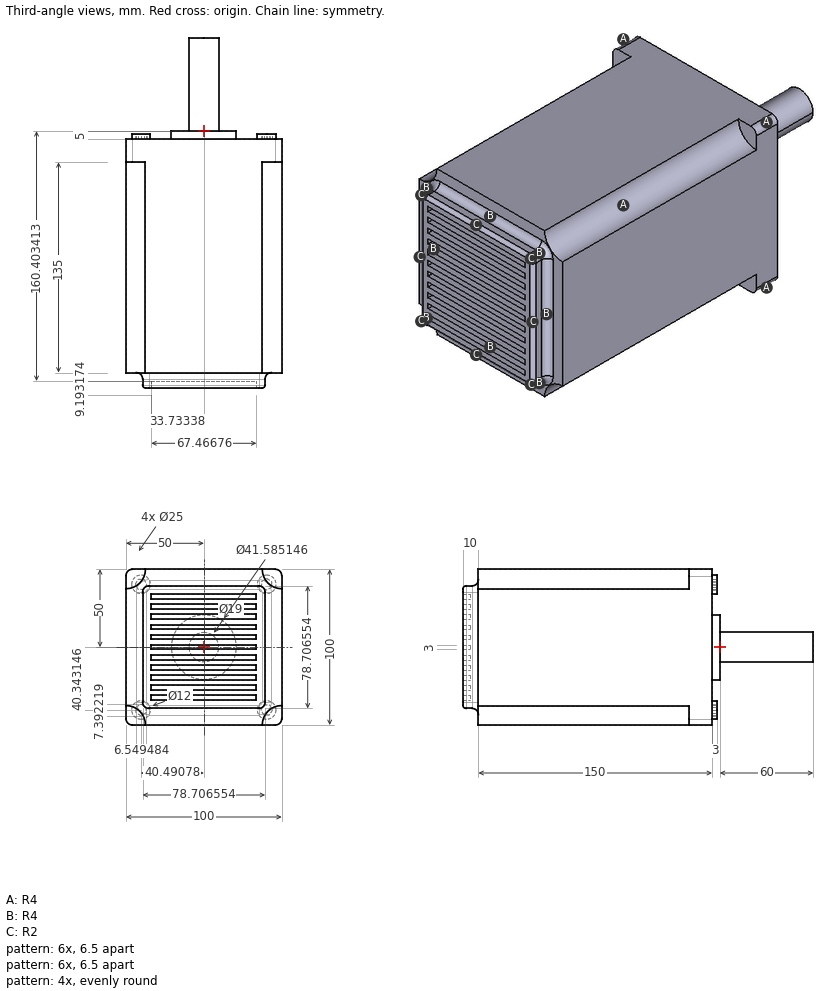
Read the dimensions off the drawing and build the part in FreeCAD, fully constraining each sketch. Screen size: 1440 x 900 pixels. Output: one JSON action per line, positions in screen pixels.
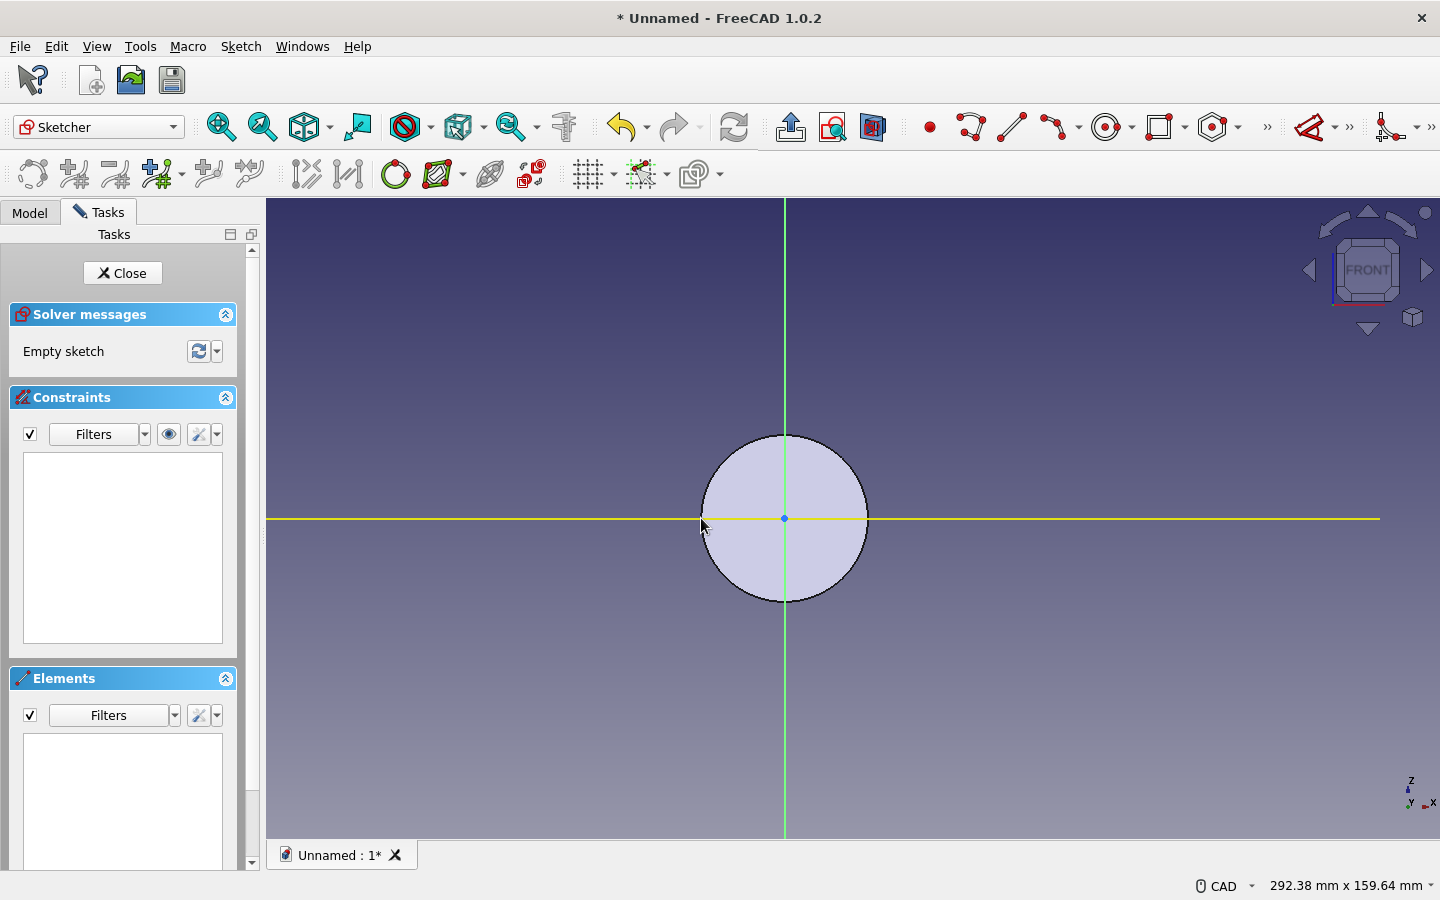
{"action": "left_click", "coordinate": [1184, 128]}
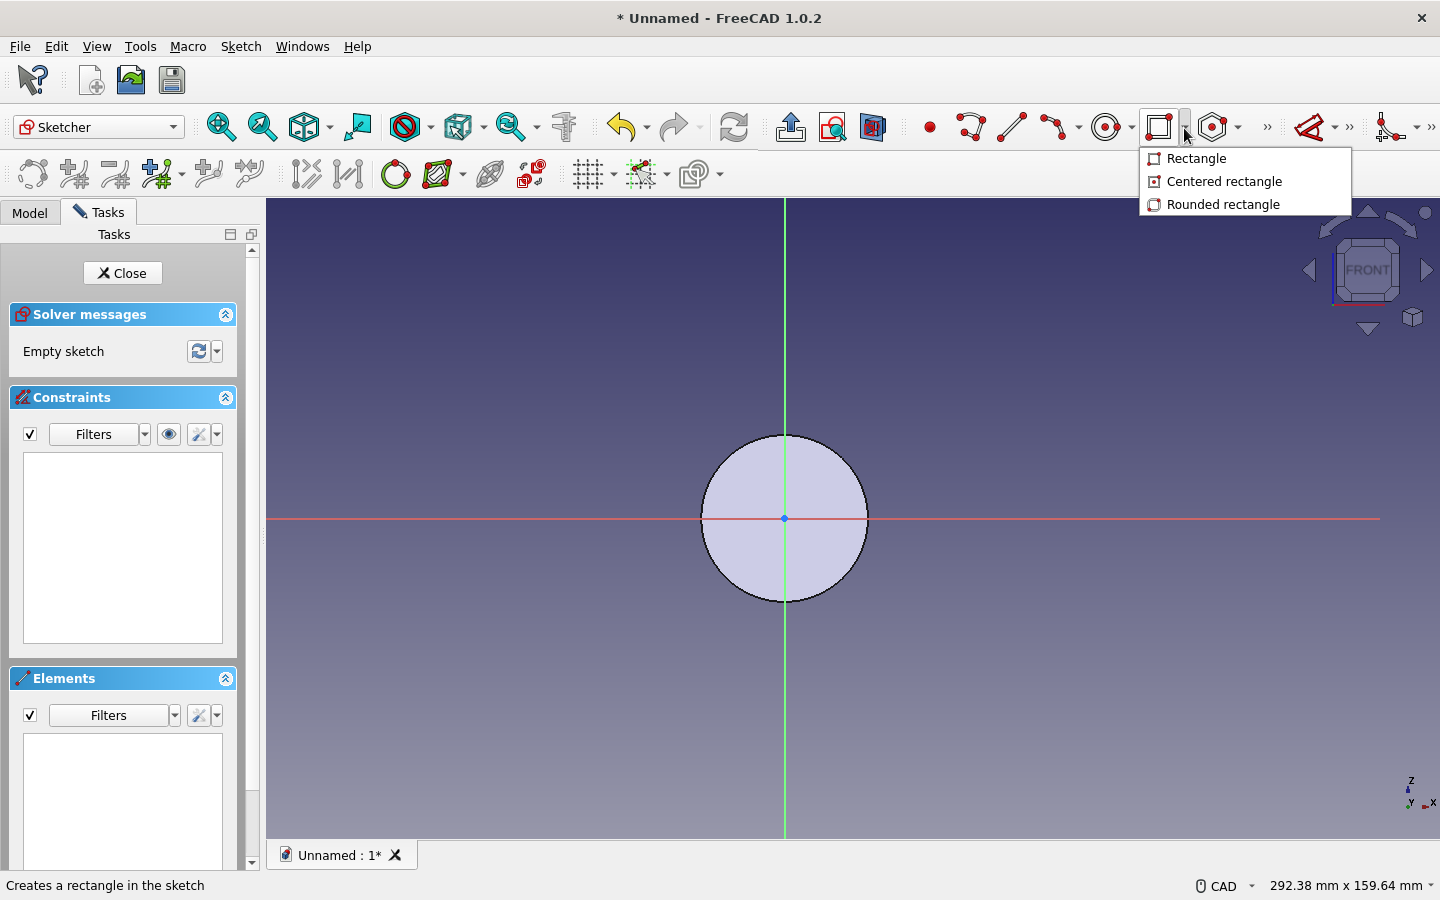
{"action": "left_click", "coordinate": [1246, 182]}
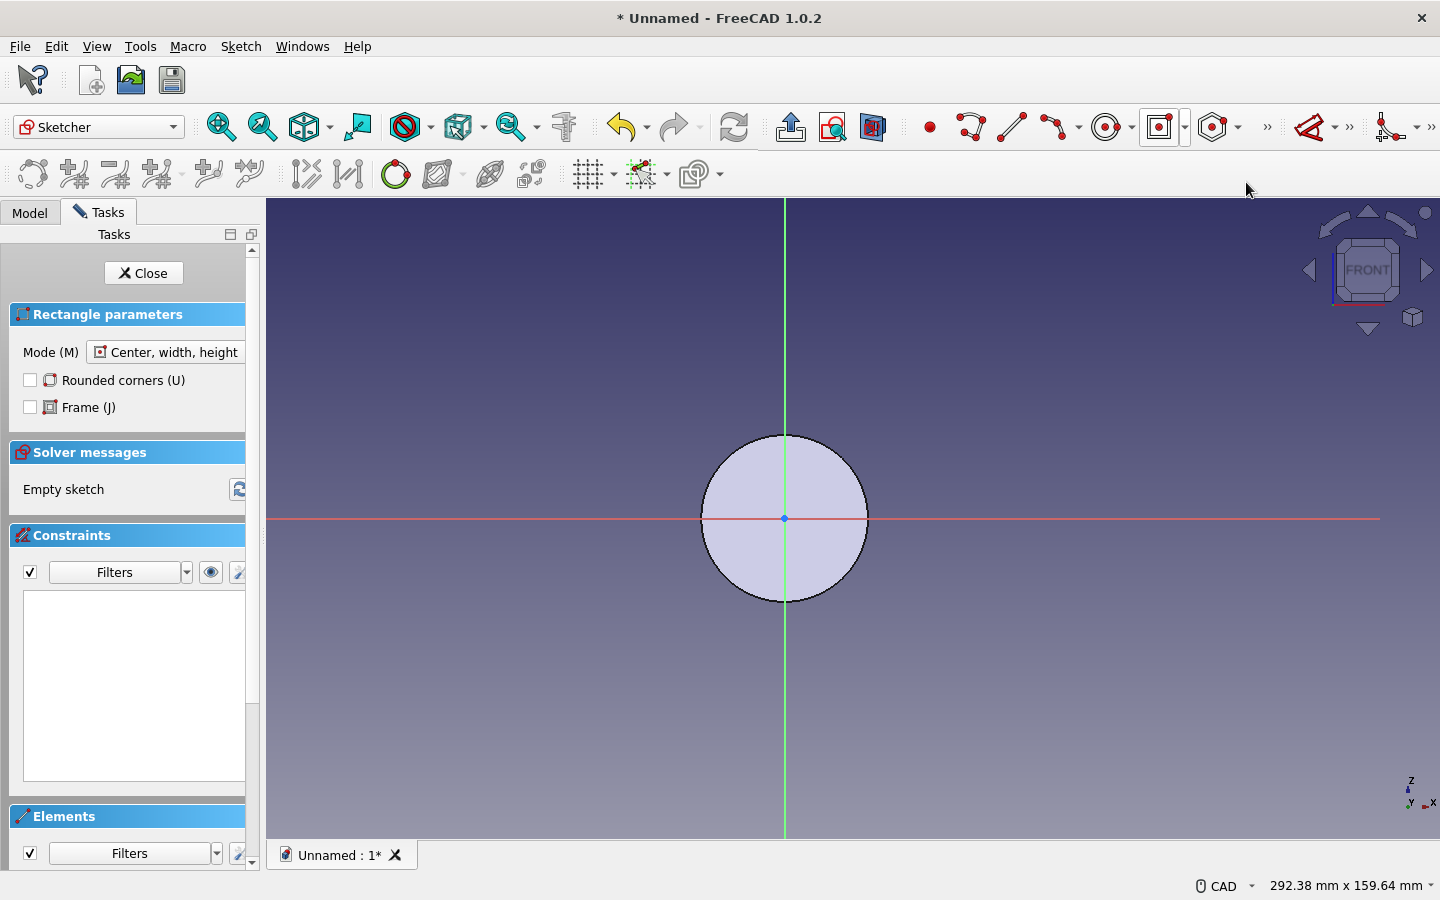
{"action": "left_click", "coordinate": [785, 519]}
{"action": "left_click", "coordinate": [985, 318]}
{"action": "key", "text": "Escape"}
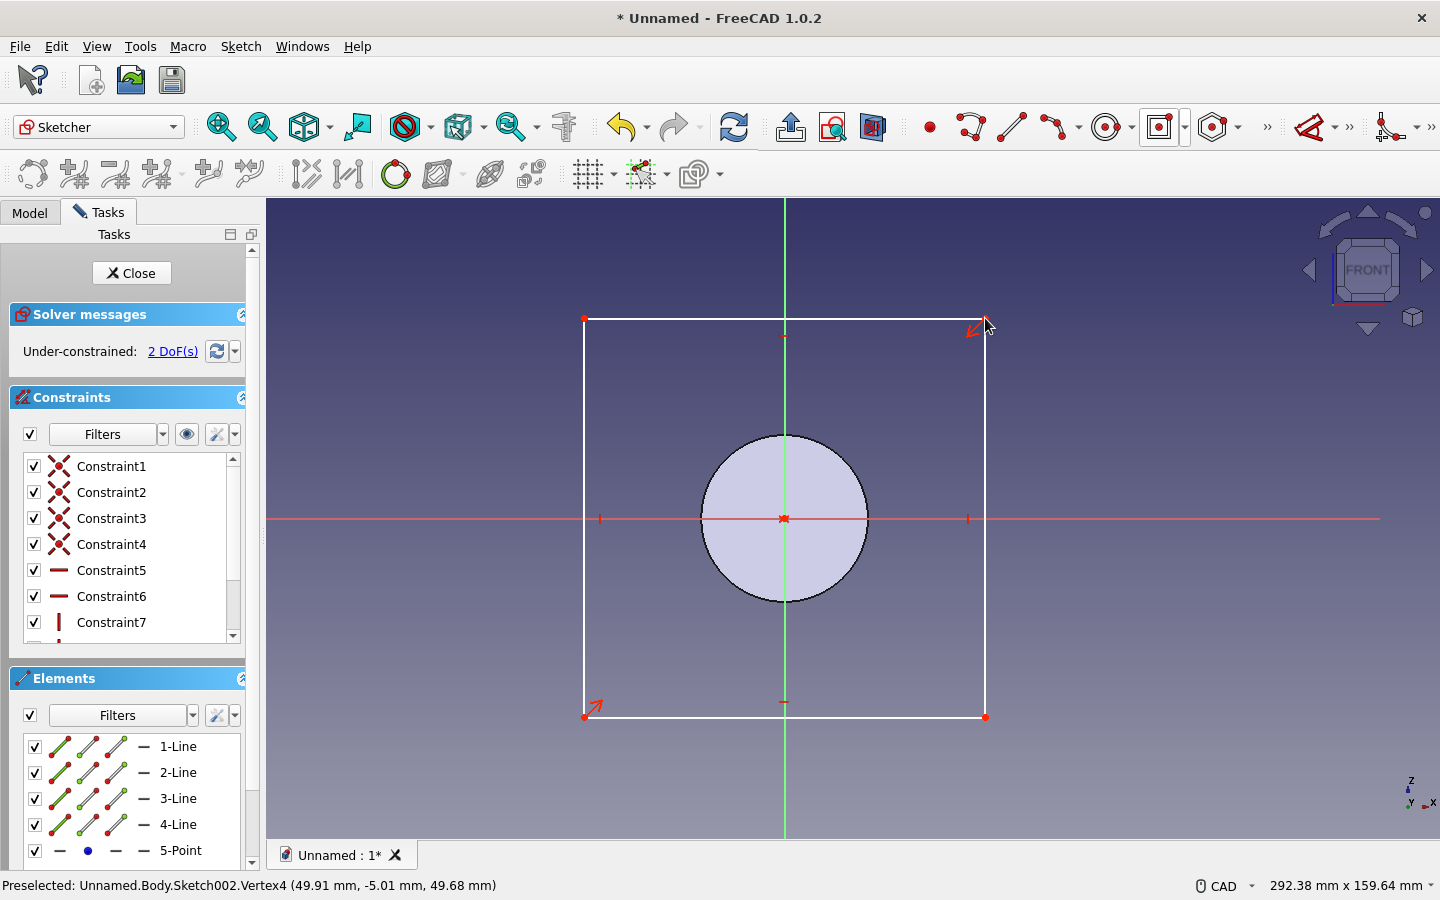
{"action": "left_click", "coordinate": [1308, 128]}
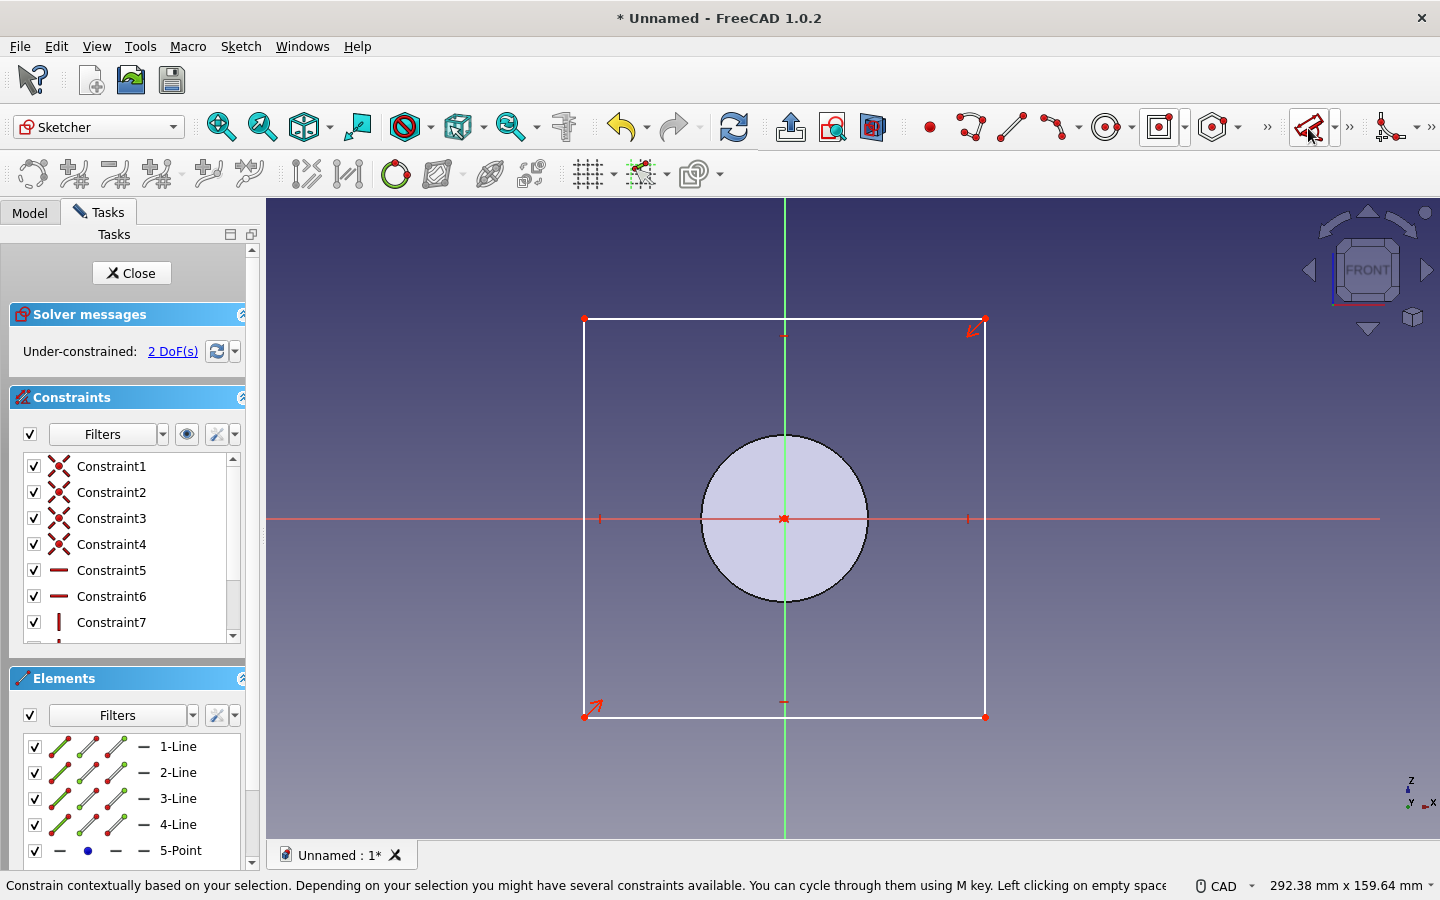
{"action": "left_click", "coordinate": [704, 718]}
{"action": "left_click", "coordinate": [692, 752]}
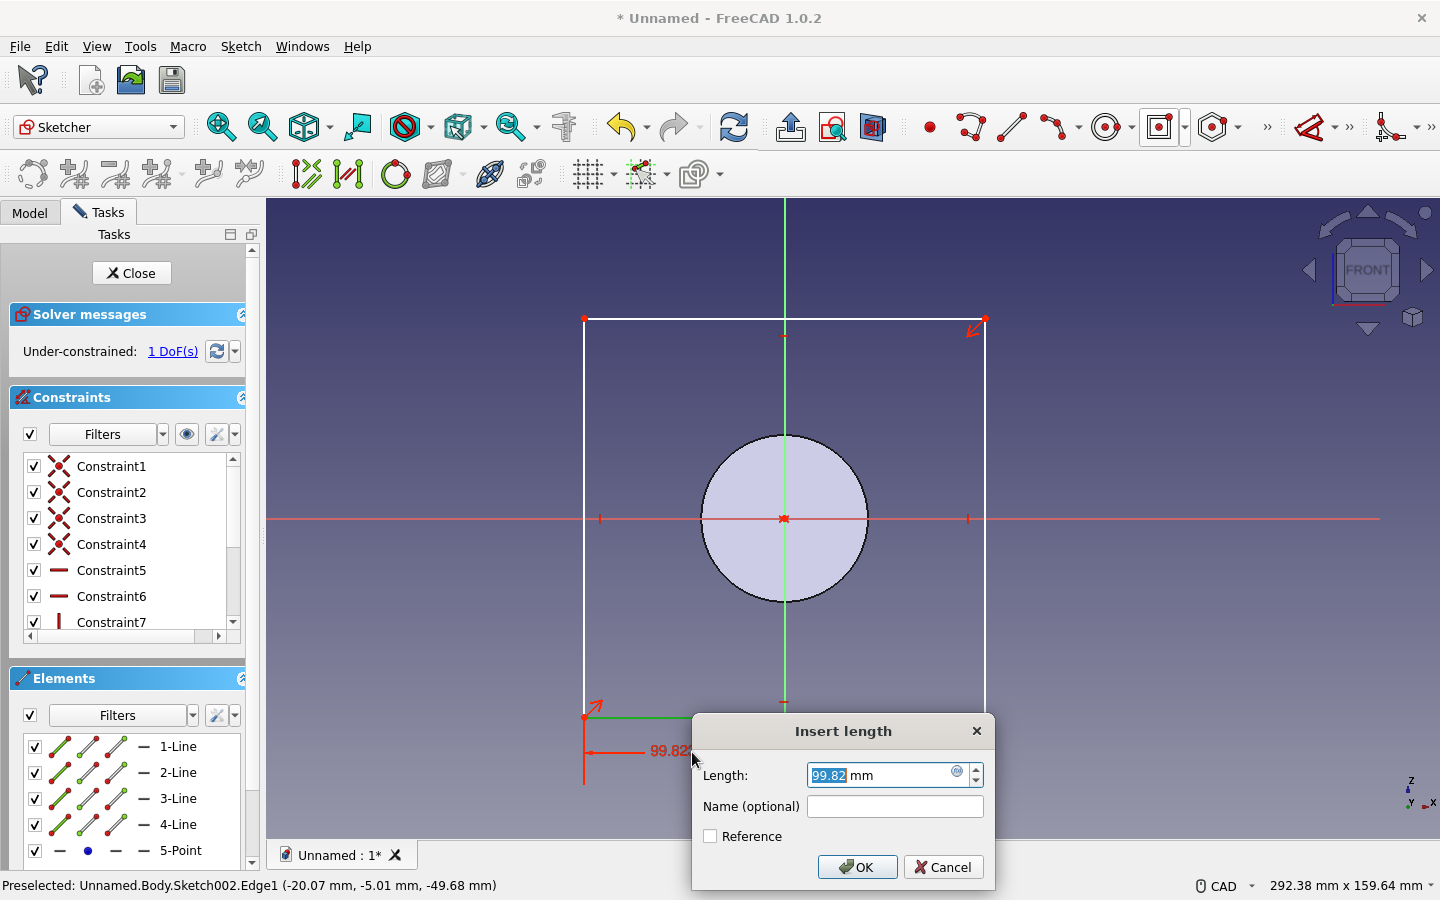
{"action": "type", "text": "100"}
{"action": "key", "text": "Return"}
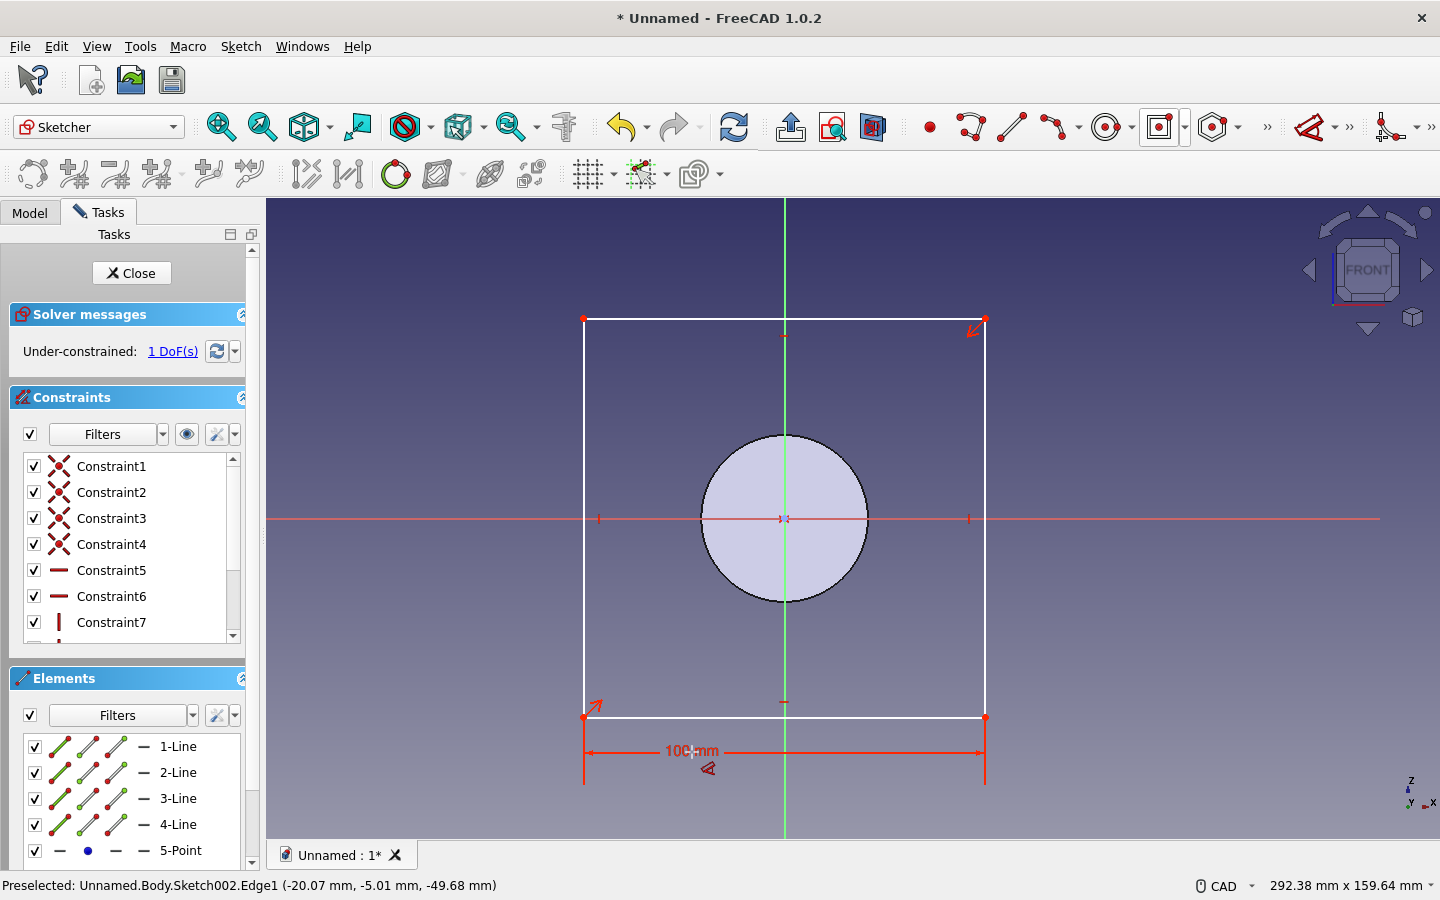
{"action": "left_click", "coordinate": [985, 598]}
{"action": "left_click", "coordinate": [1019, 427]}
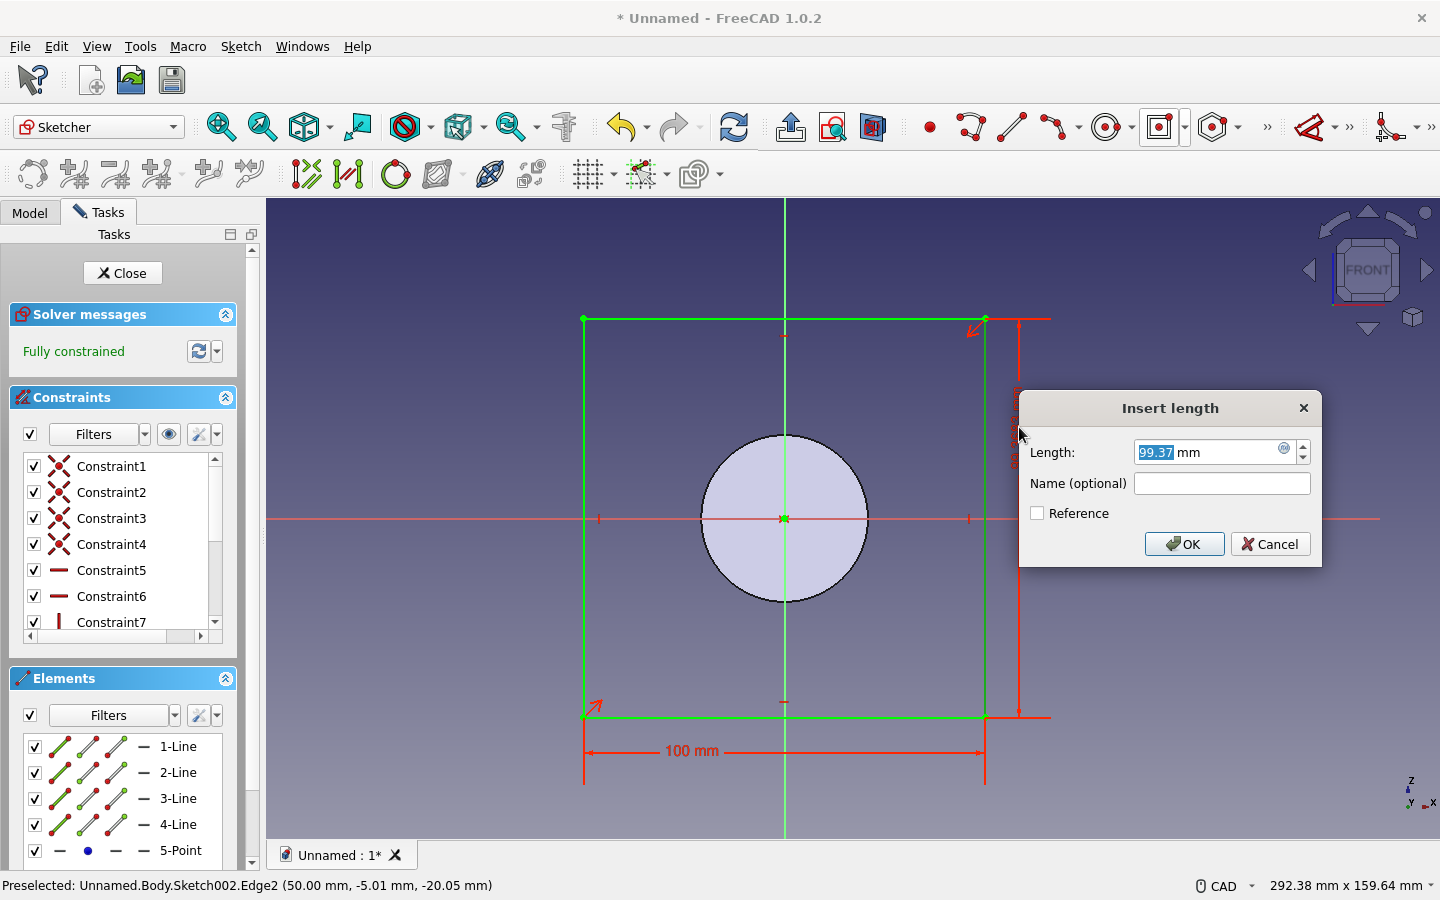
{"action": "type", "text": "100"}
{"action": "key", "text": "Return"}
{"action": "key", "text": "Escape"}